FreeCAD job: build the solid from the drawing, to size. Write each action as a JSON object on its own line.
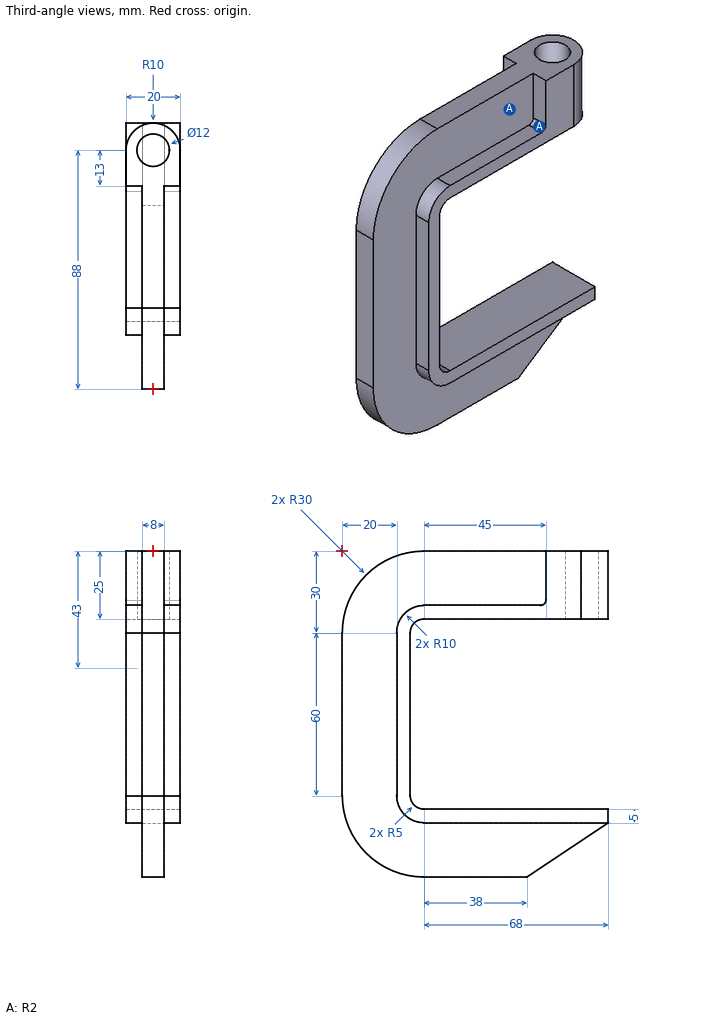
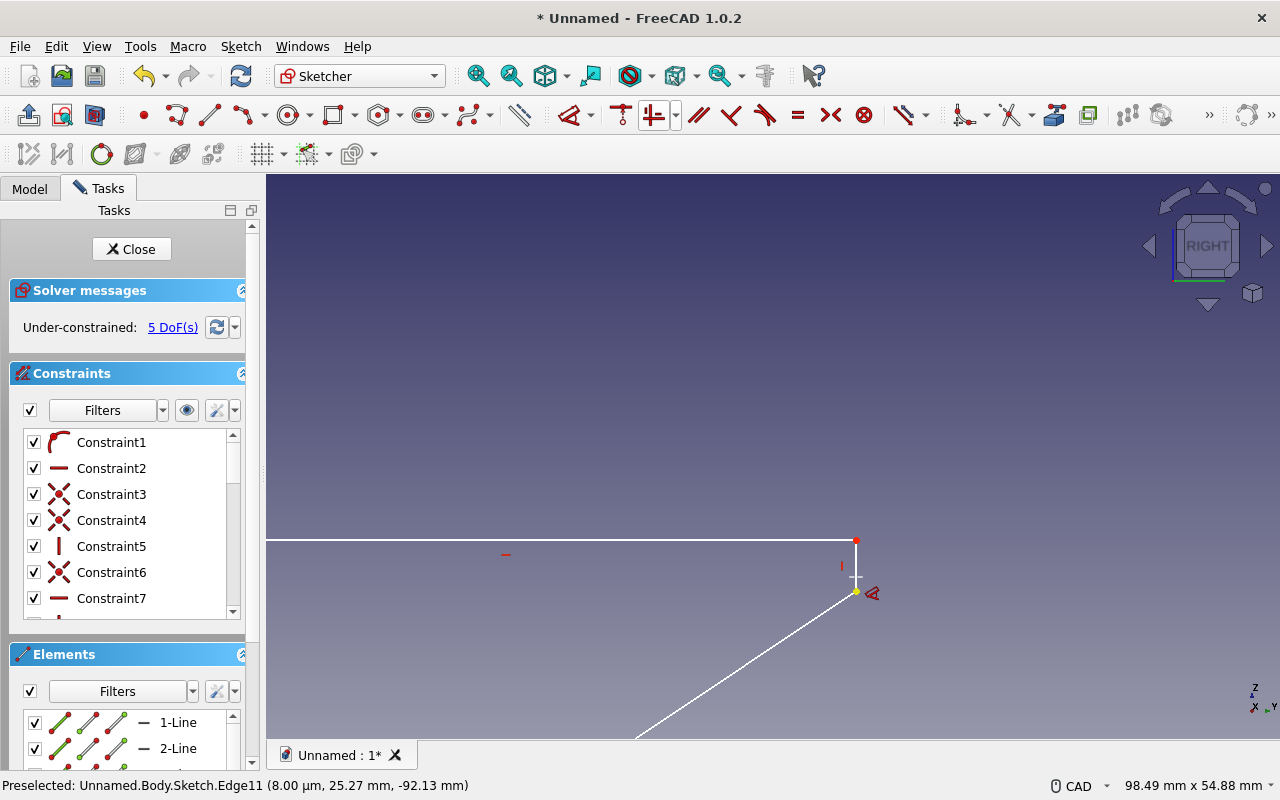
{"action": "left_click", "coordinate": [856, 576]}
{"action": "left_click", "coordinate": [890, 566]}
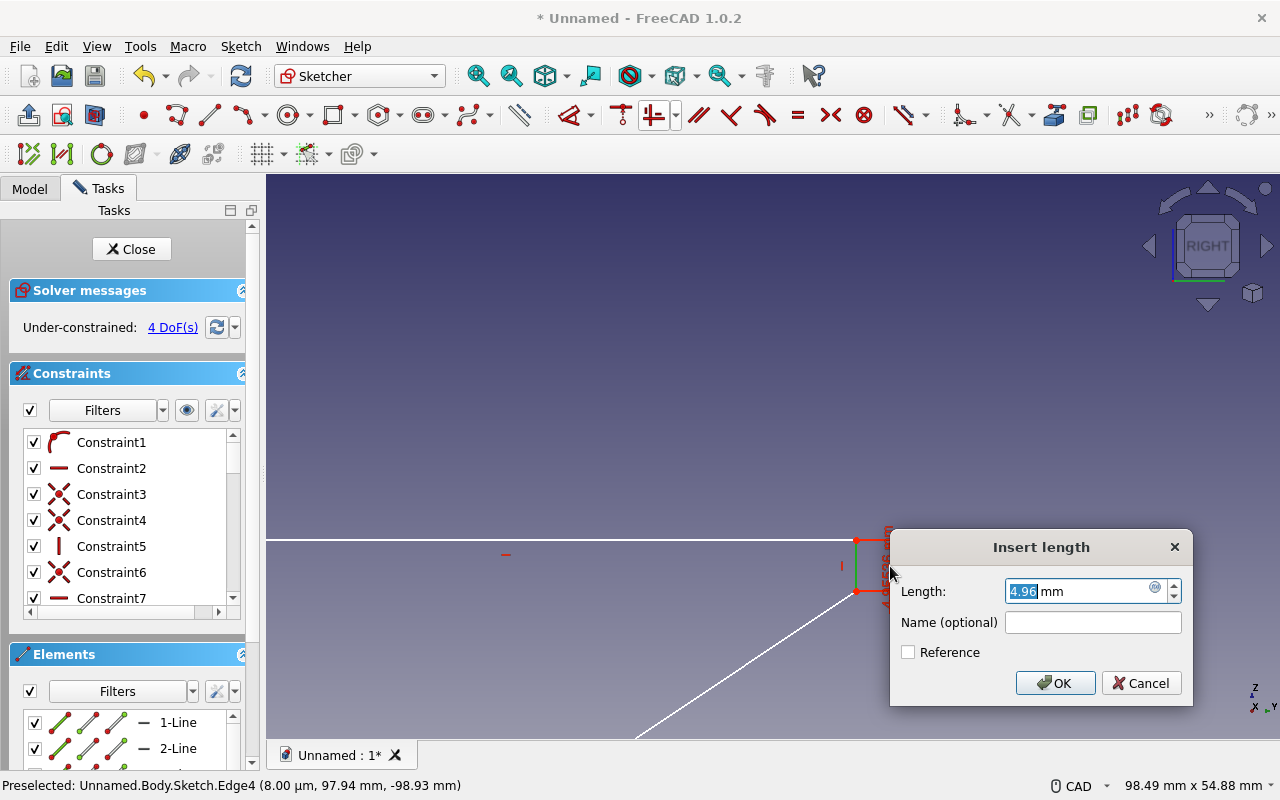
{"action": "type", "text": "5"}
{"action": "key", "text": "Return"}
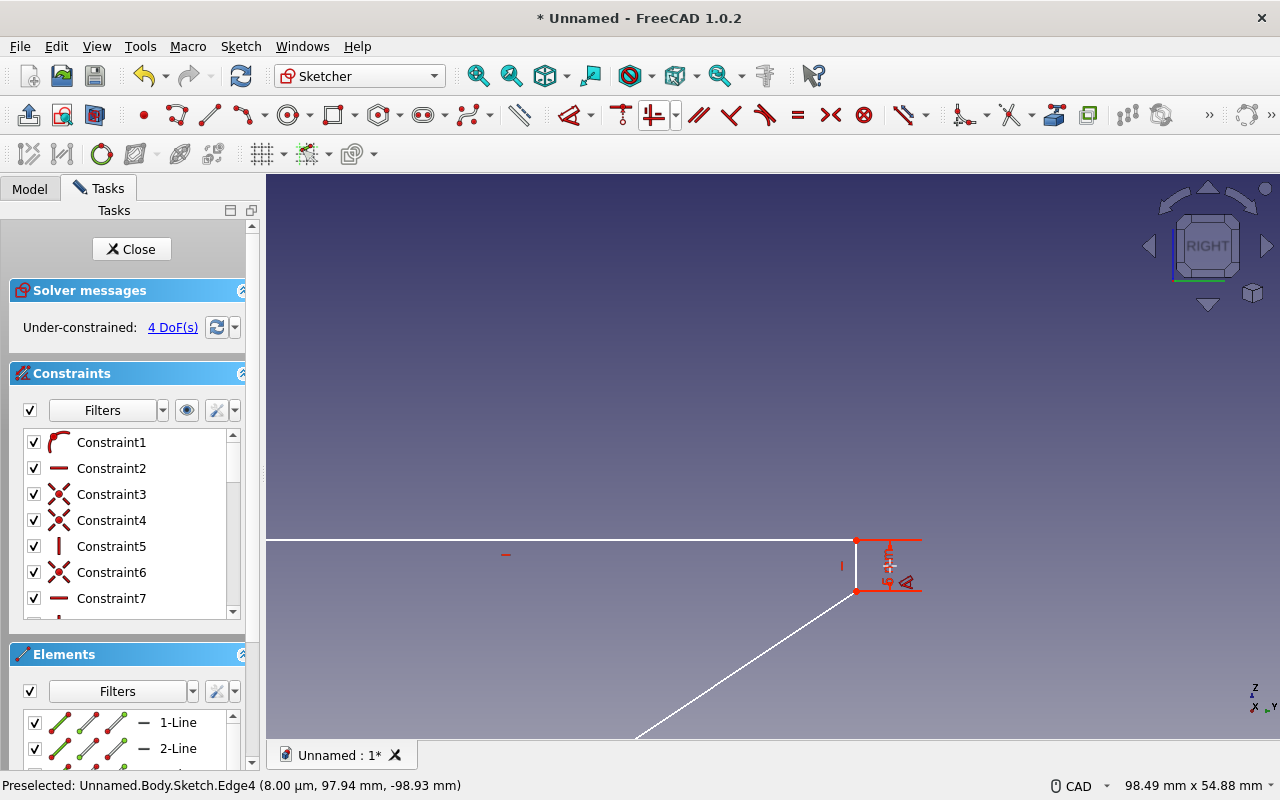
{"action": "scroll", "coordinate": [856, 577], "scroll_direction": "down", "scroll_amount": 6}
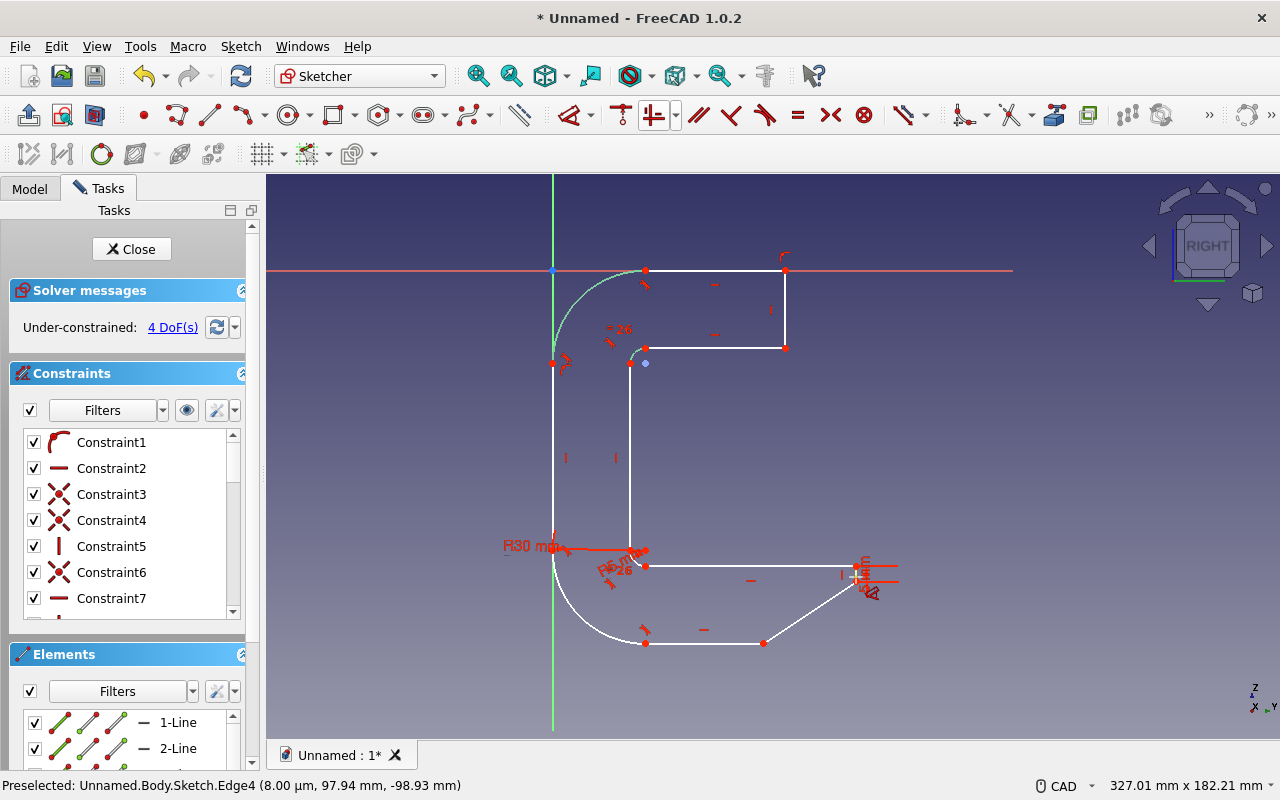
{"action": "left_click", "coordinate": [553, 420]}
{"action": "left_click", "coordinate": [519, 457]}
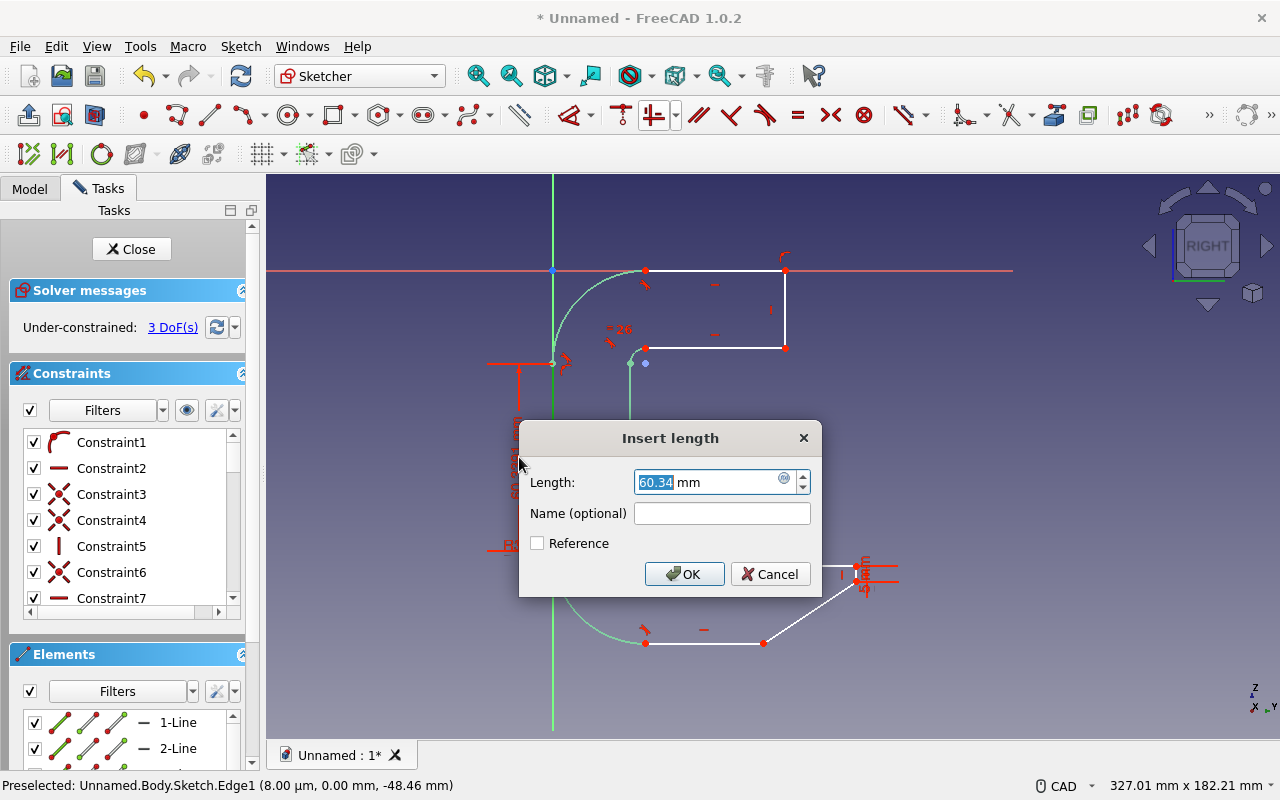
{"action": "type", "text": "60"}
{"action": "key", "text": "Return"}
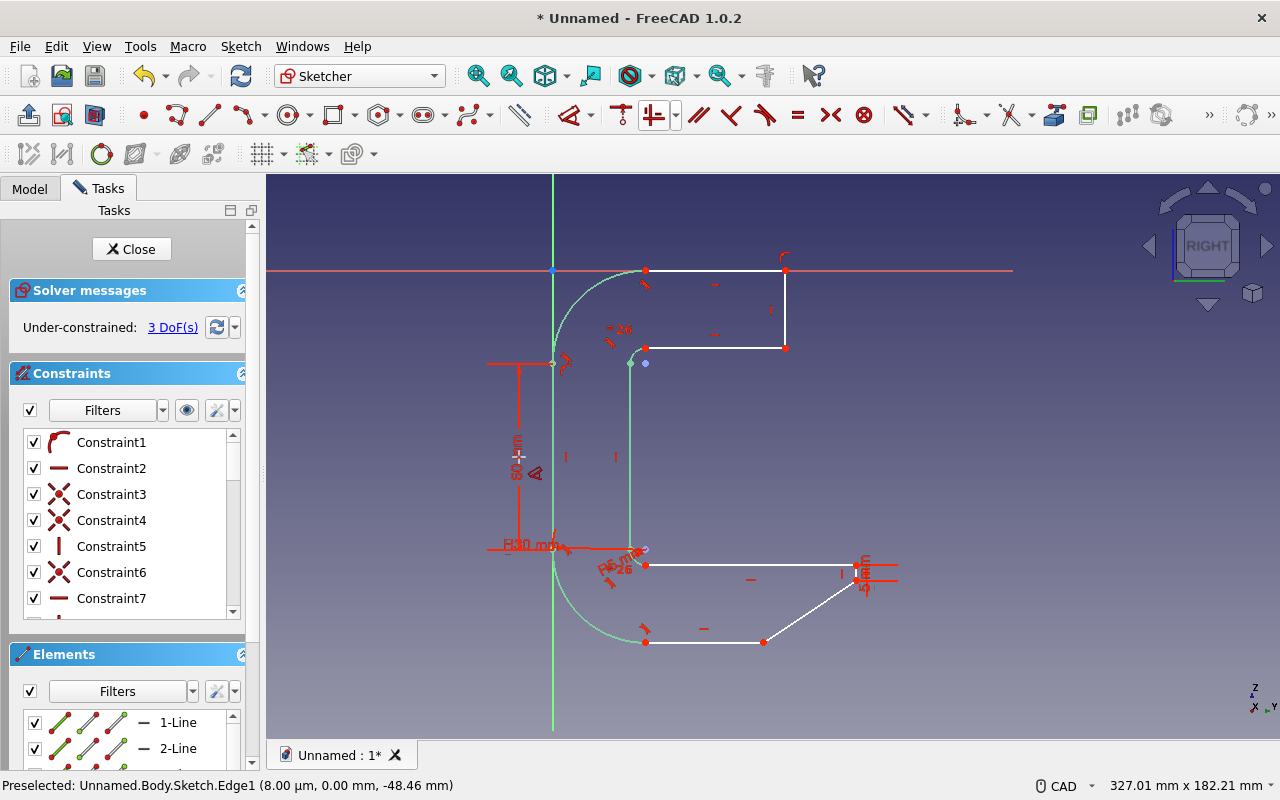
{"action": "left_click", "coordinate": [681, 643]}
{"action": "left_click", "coordinate": [705, 677]}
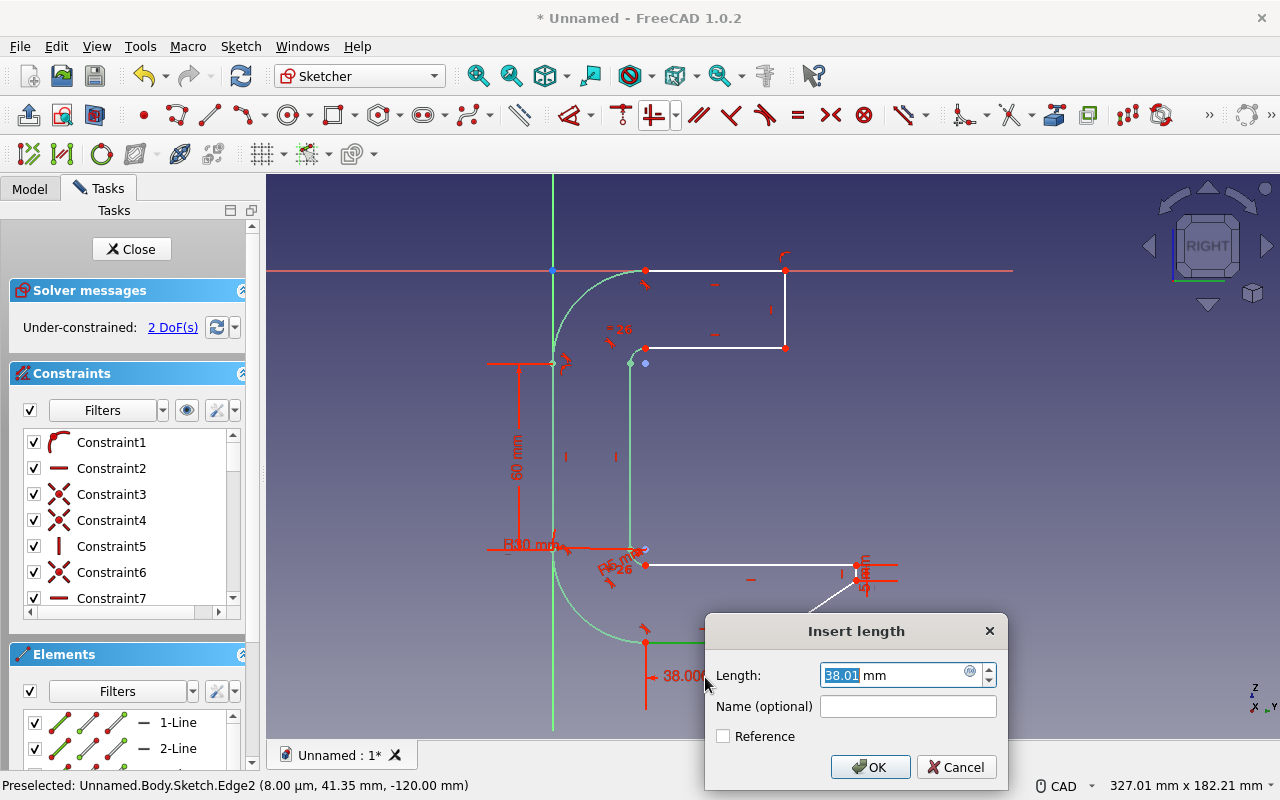
{"action": "type", "text": "38"}
{"action": "key", "text": "Return"}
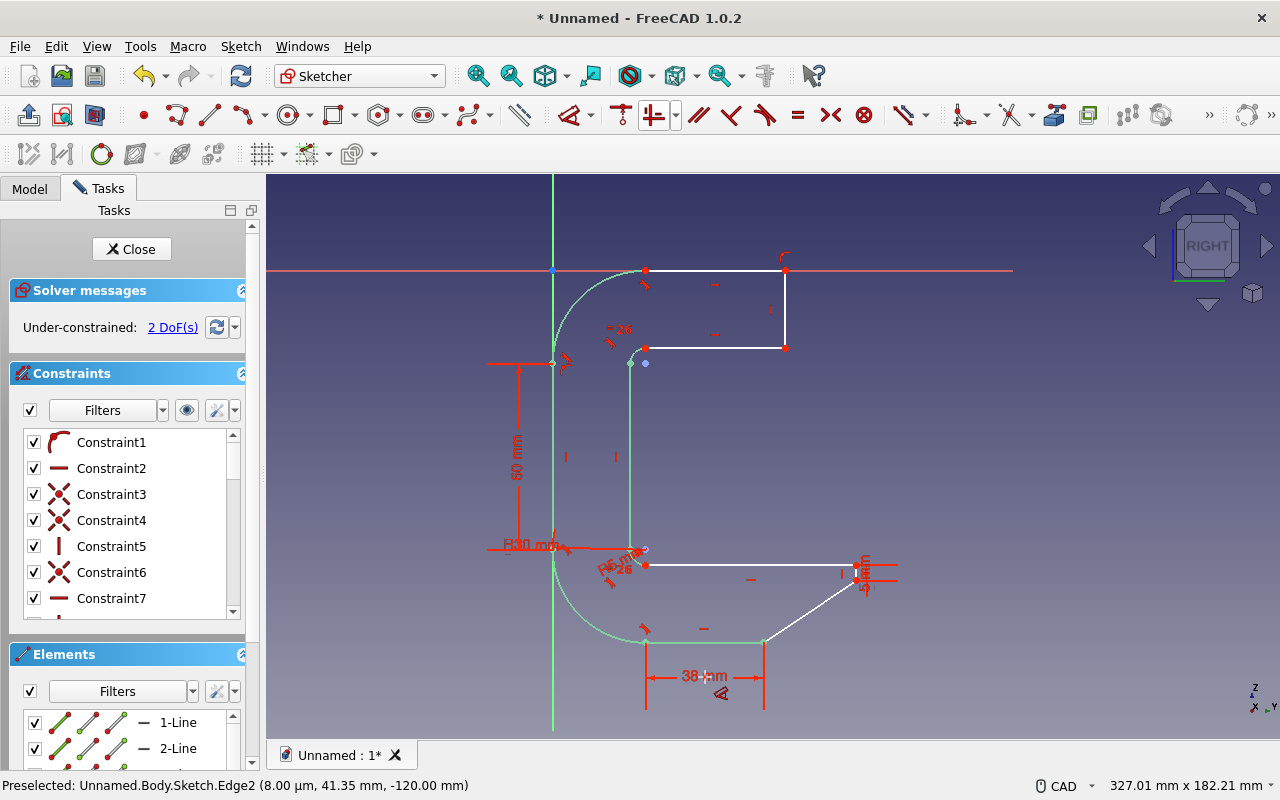
{"action": "left_click", "coordinate": [793, 565]}
{"action": "left_click", "coordinate": [751, 599]}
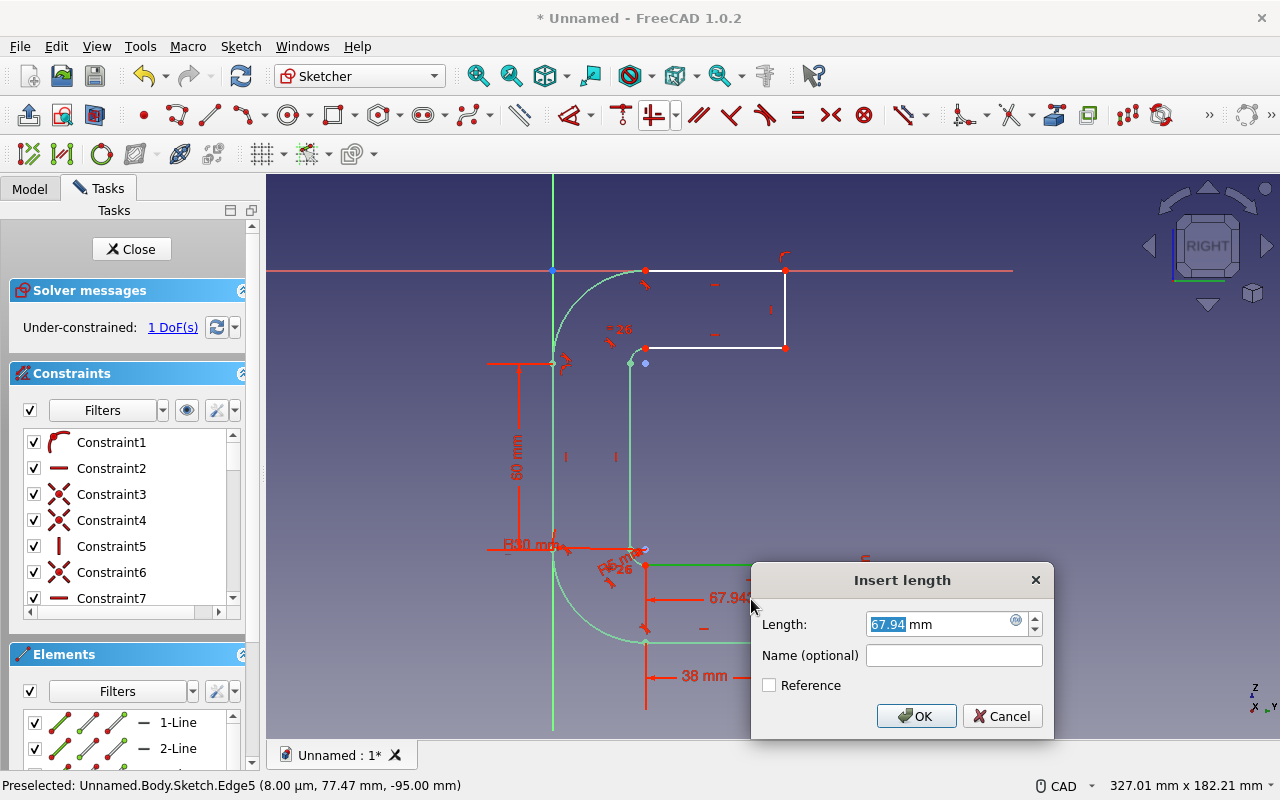
{"action": "type", "text": "68"}
{"action": "key", "text": "Return"}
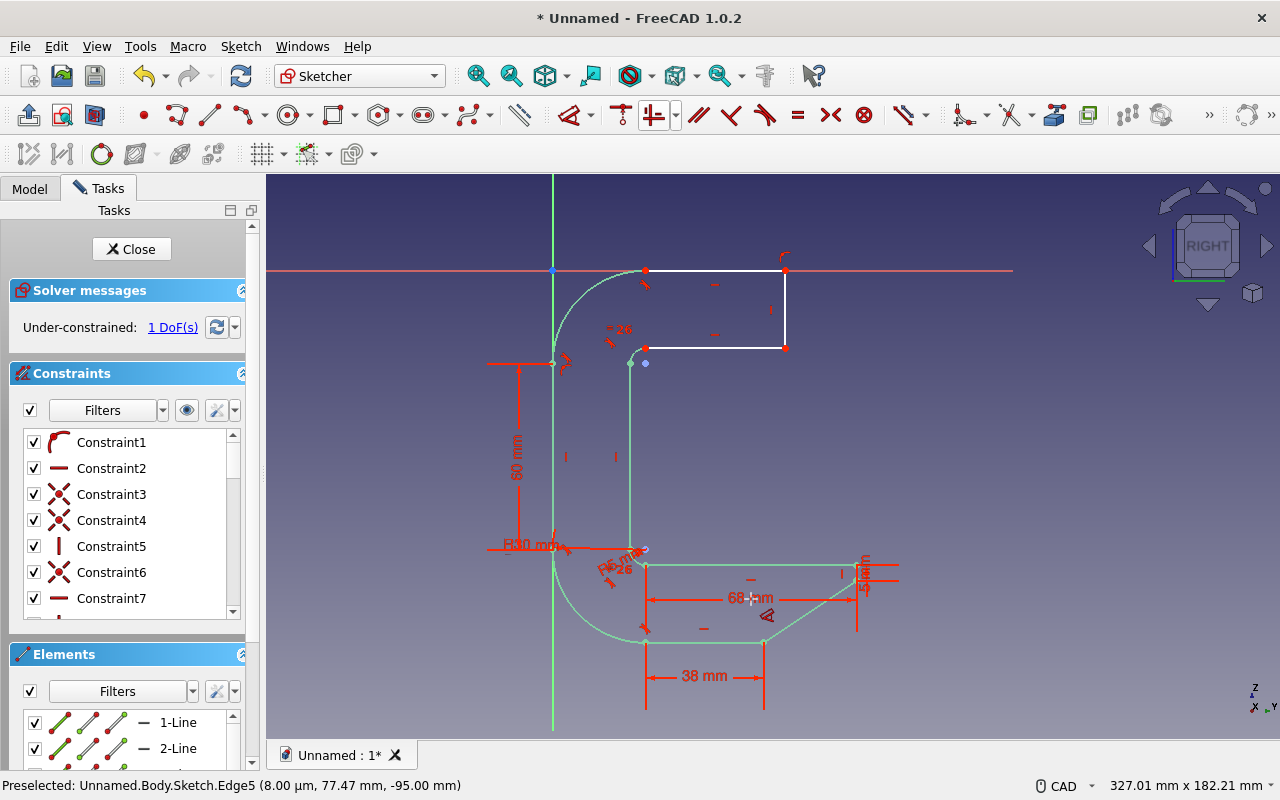
{"action": "left_click", "coordinate": [688, 348]}
{"action": "left_click", "coordinate": [716, 314]}